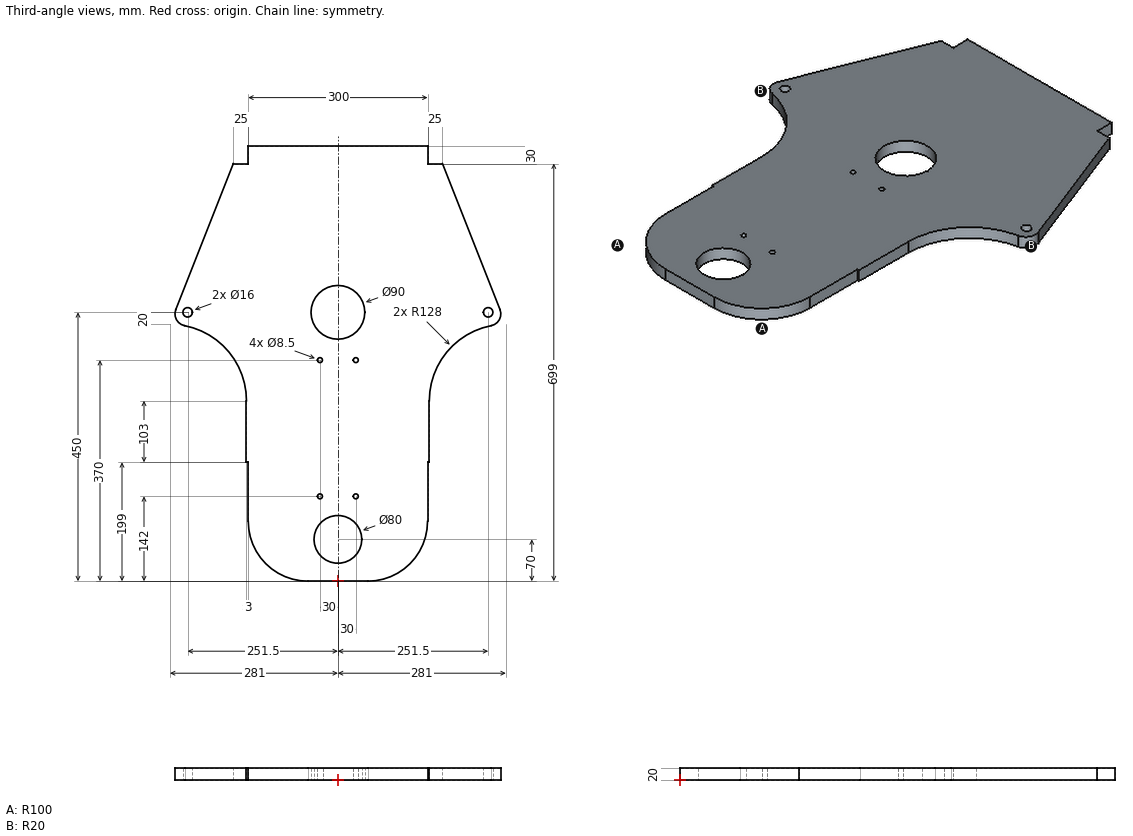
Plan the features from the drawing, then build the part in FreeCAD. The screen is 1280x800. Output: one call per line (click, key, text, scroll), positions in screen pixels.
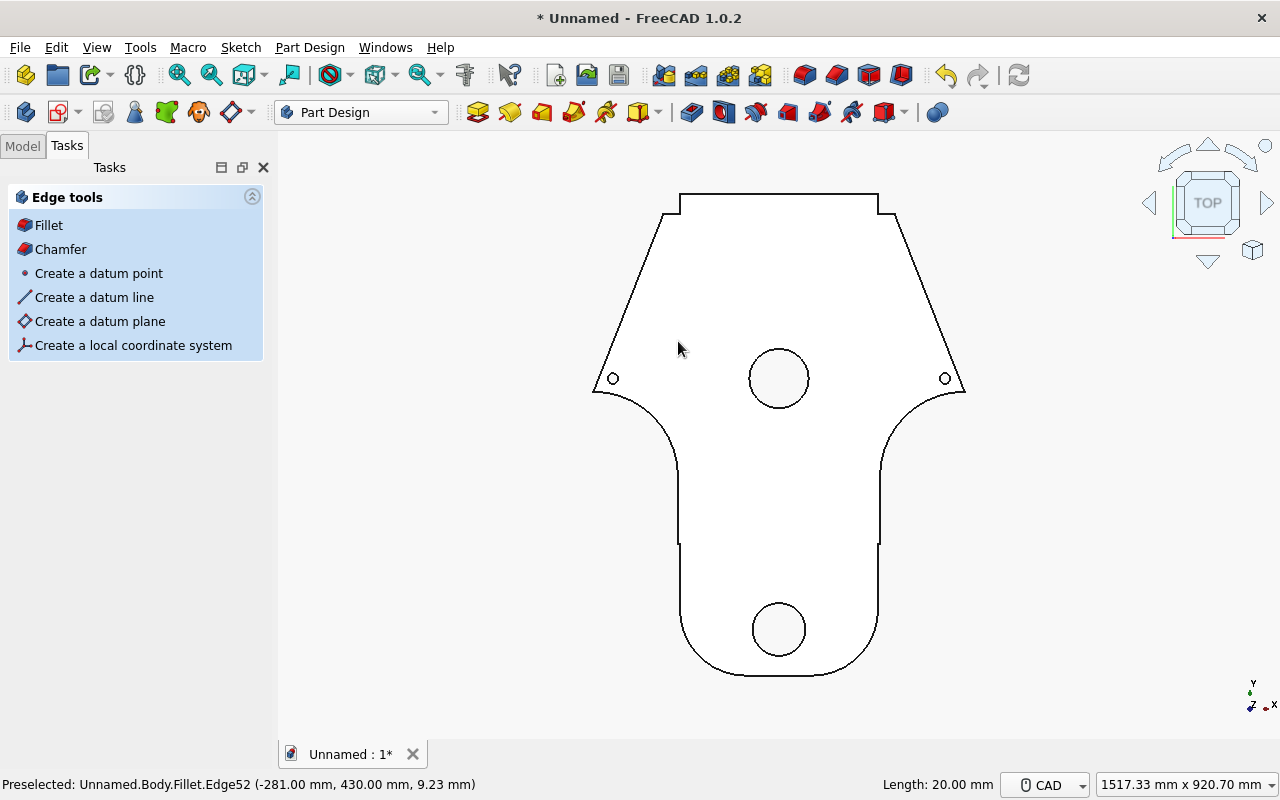
scroll(593, 391, up, 6)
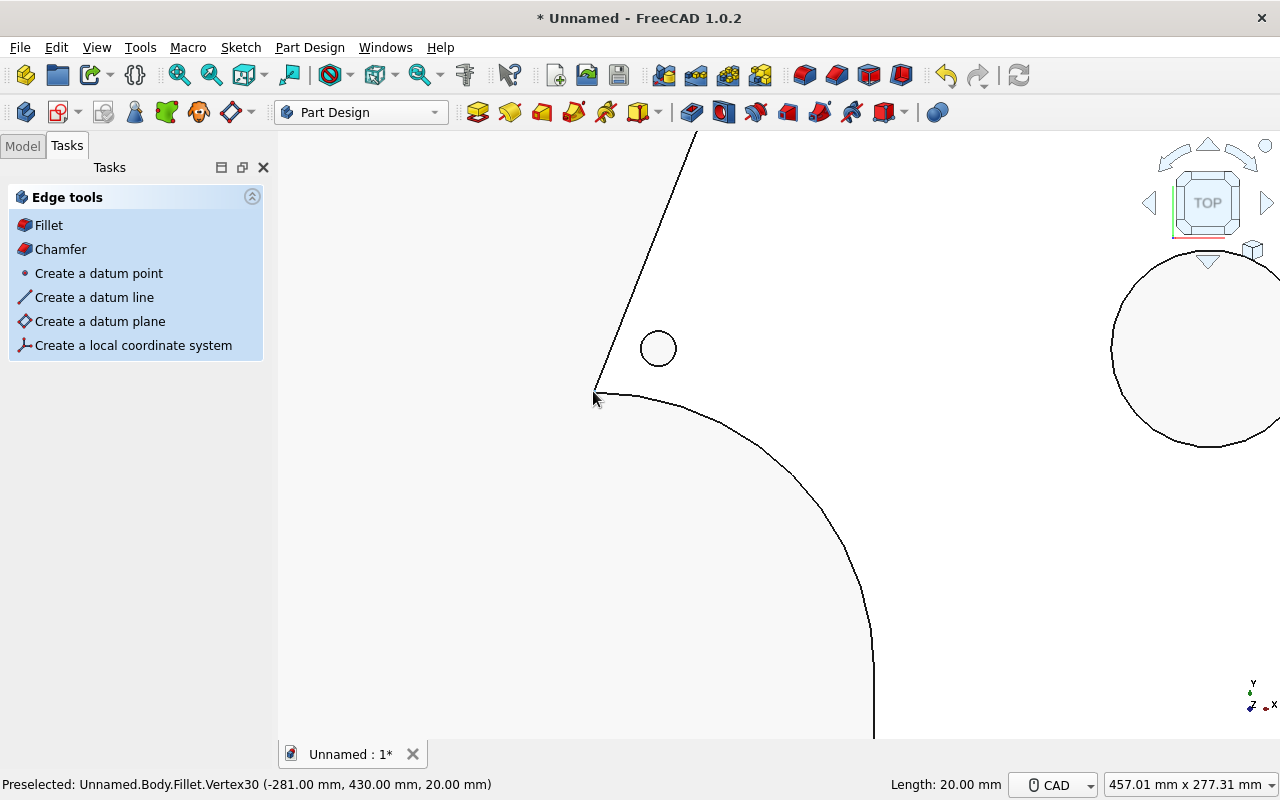
click(180, 76)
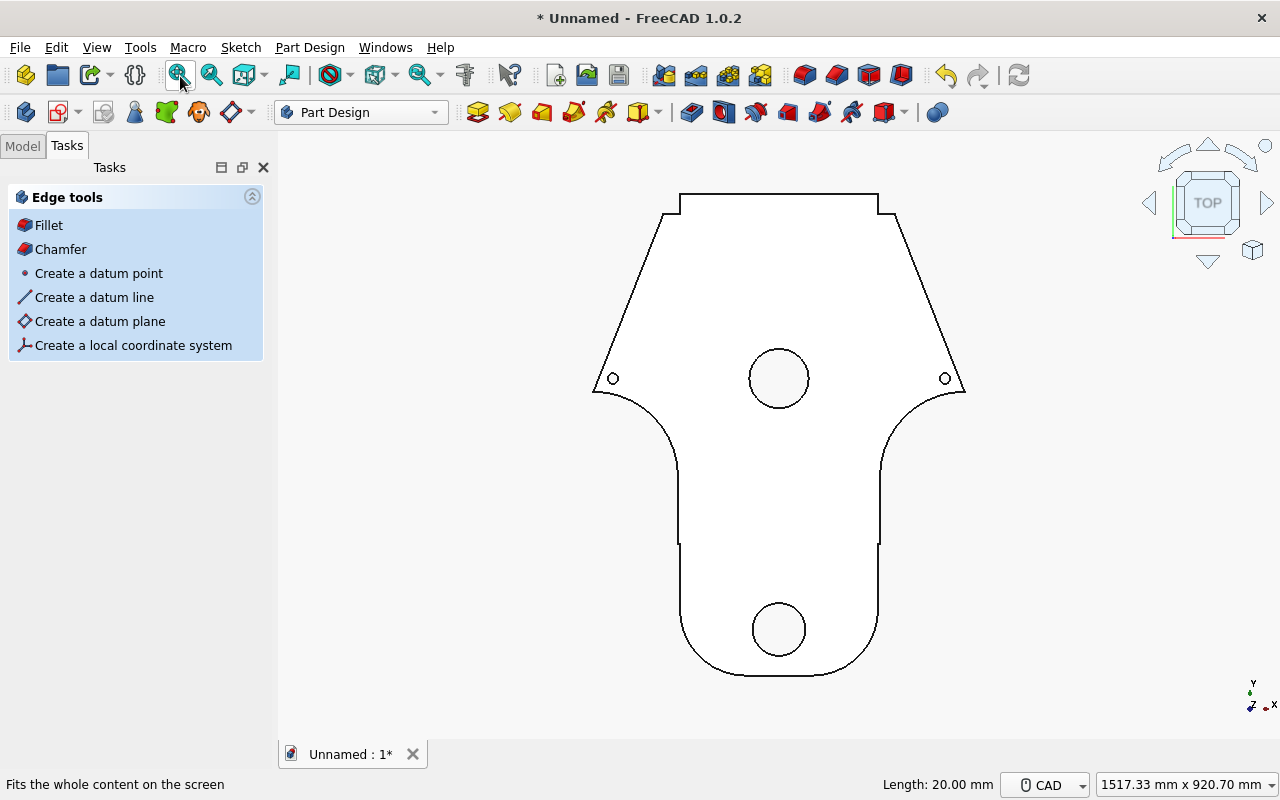
key(1)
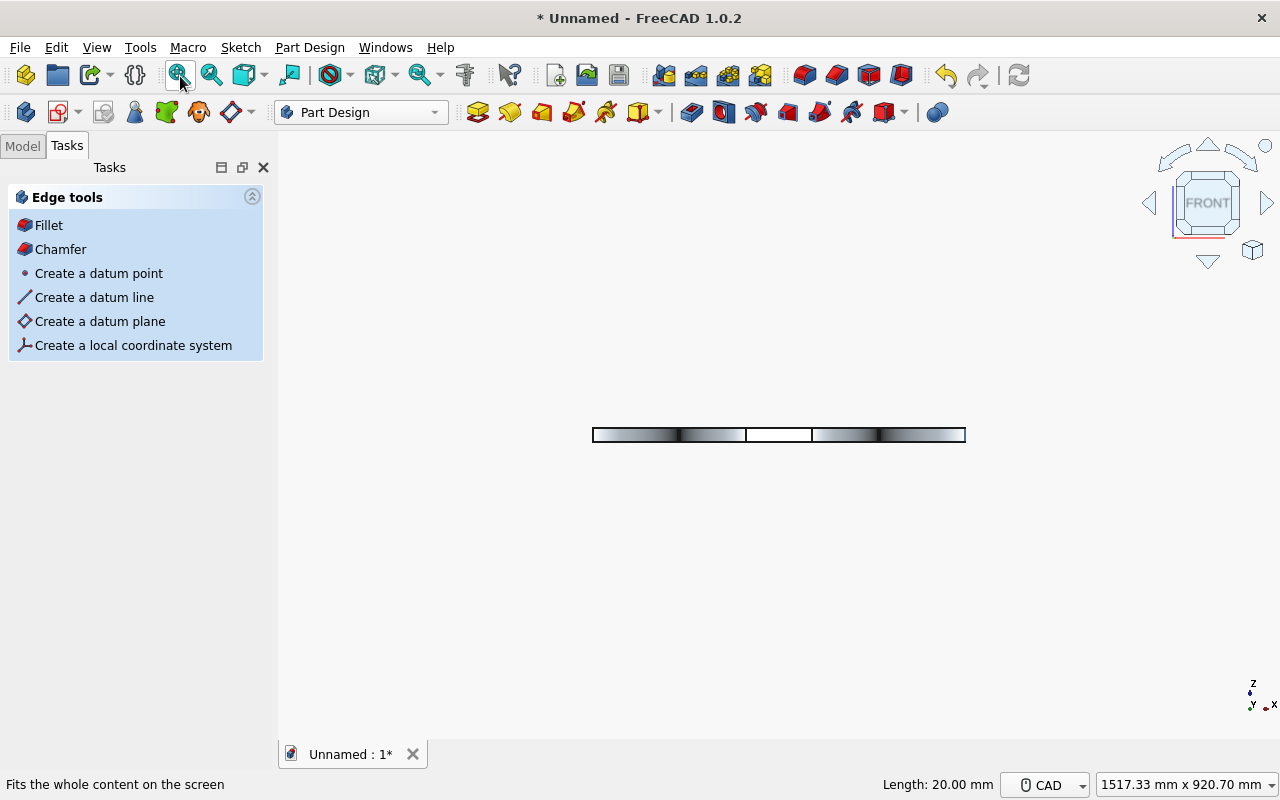
click(180, 76)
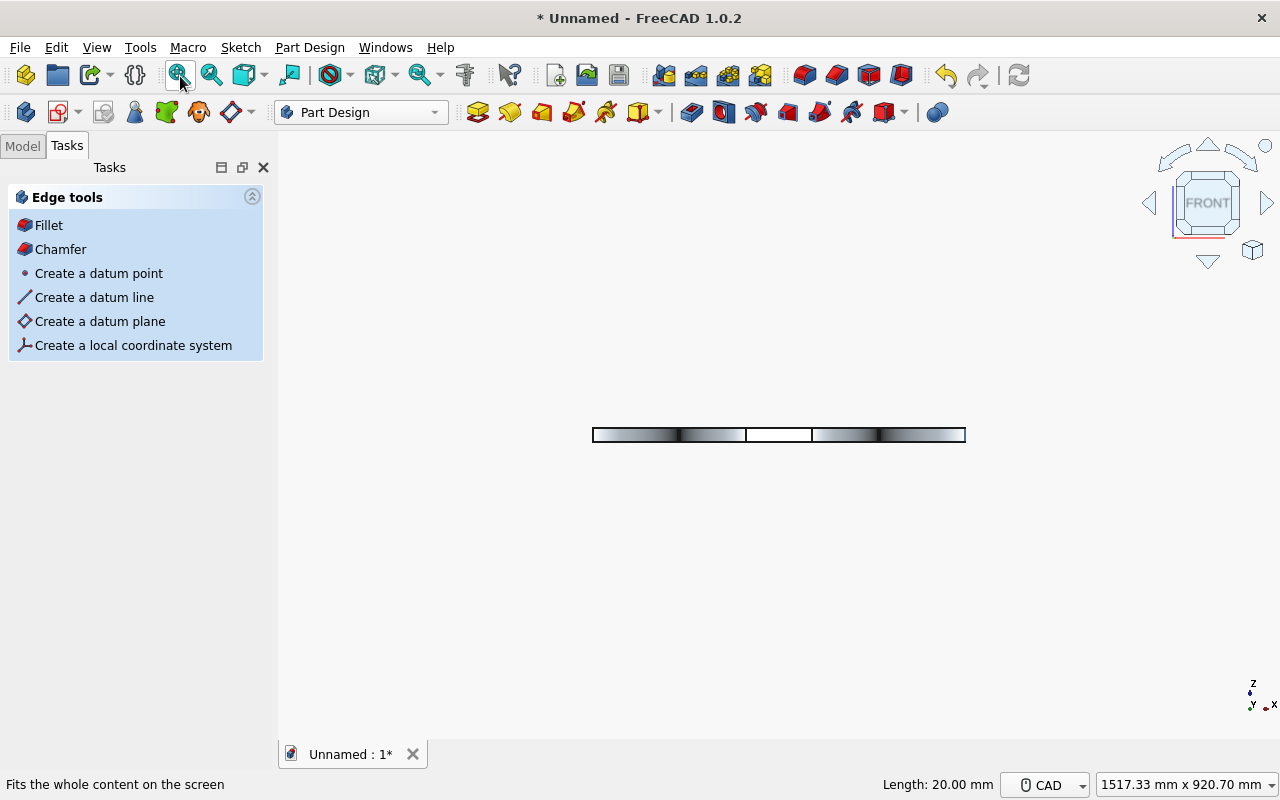
scroll(593, 434, up, 6)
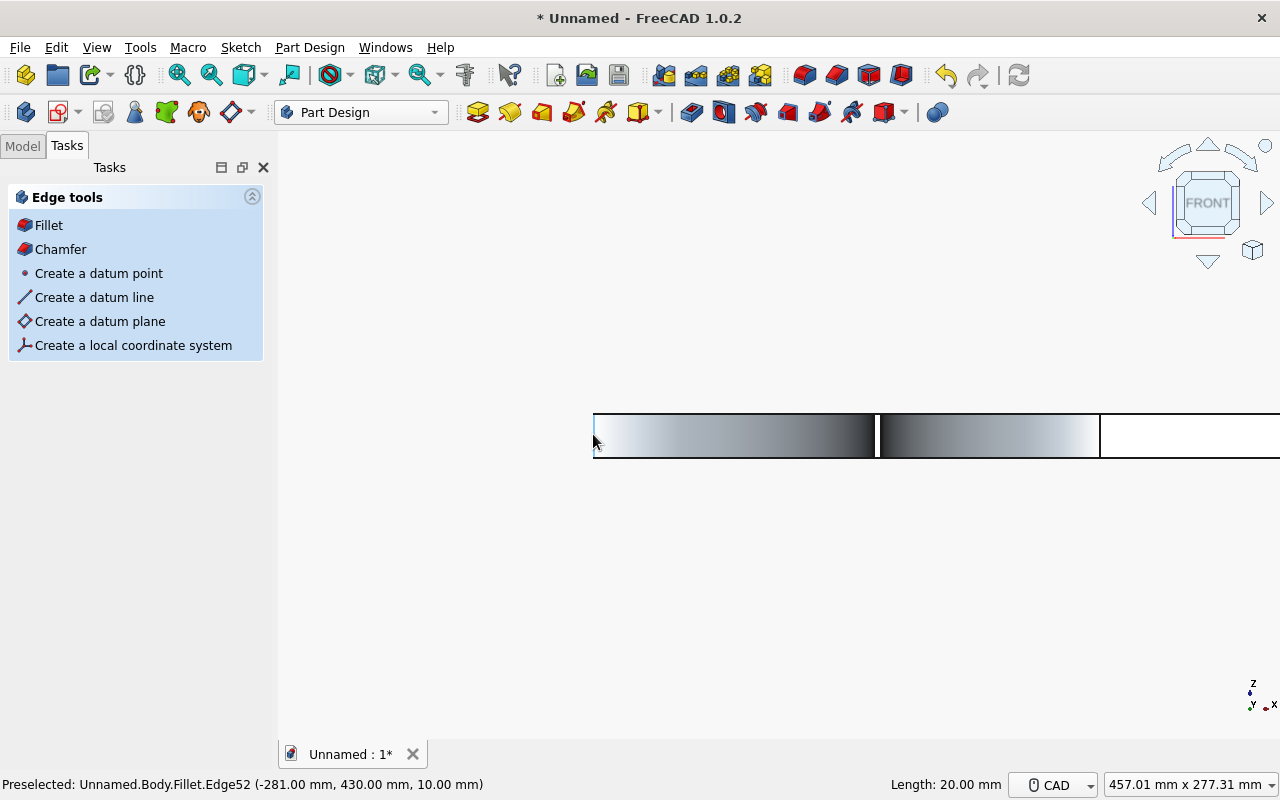
click(180, 76)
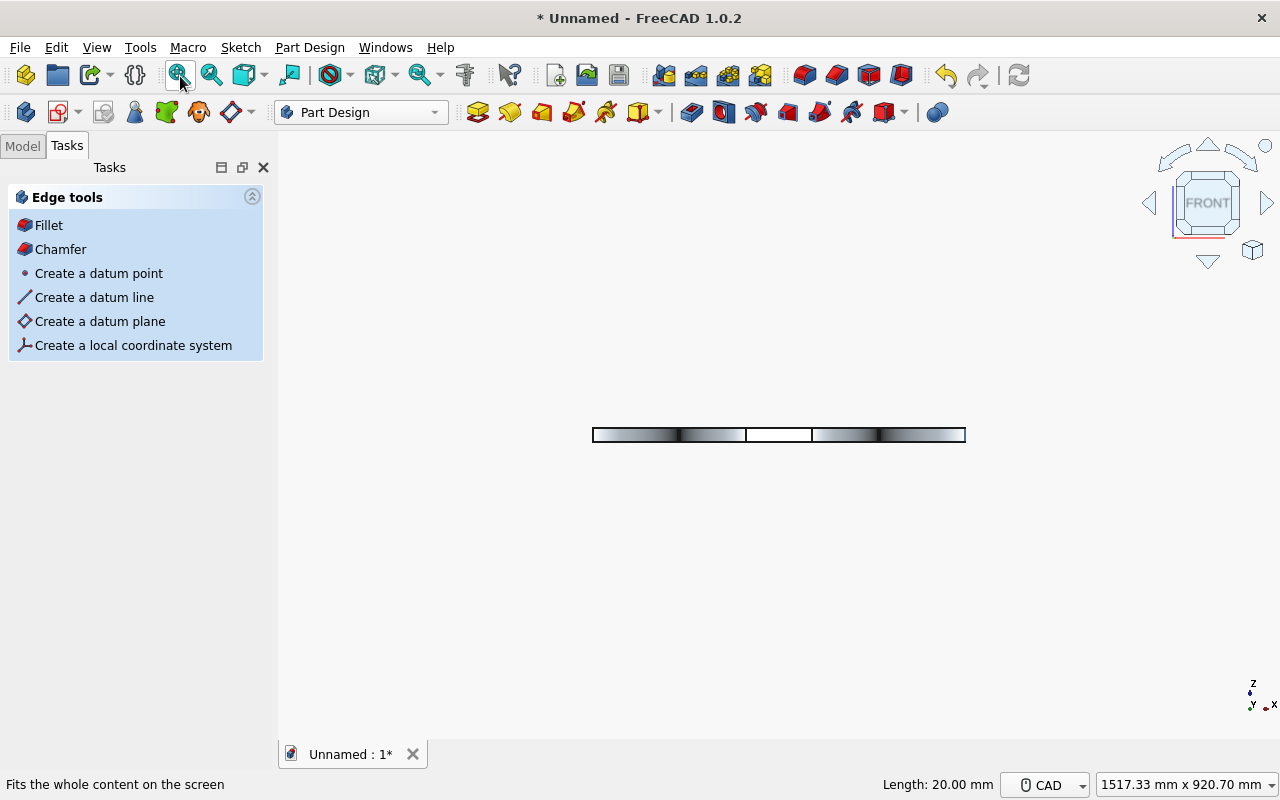
key(3)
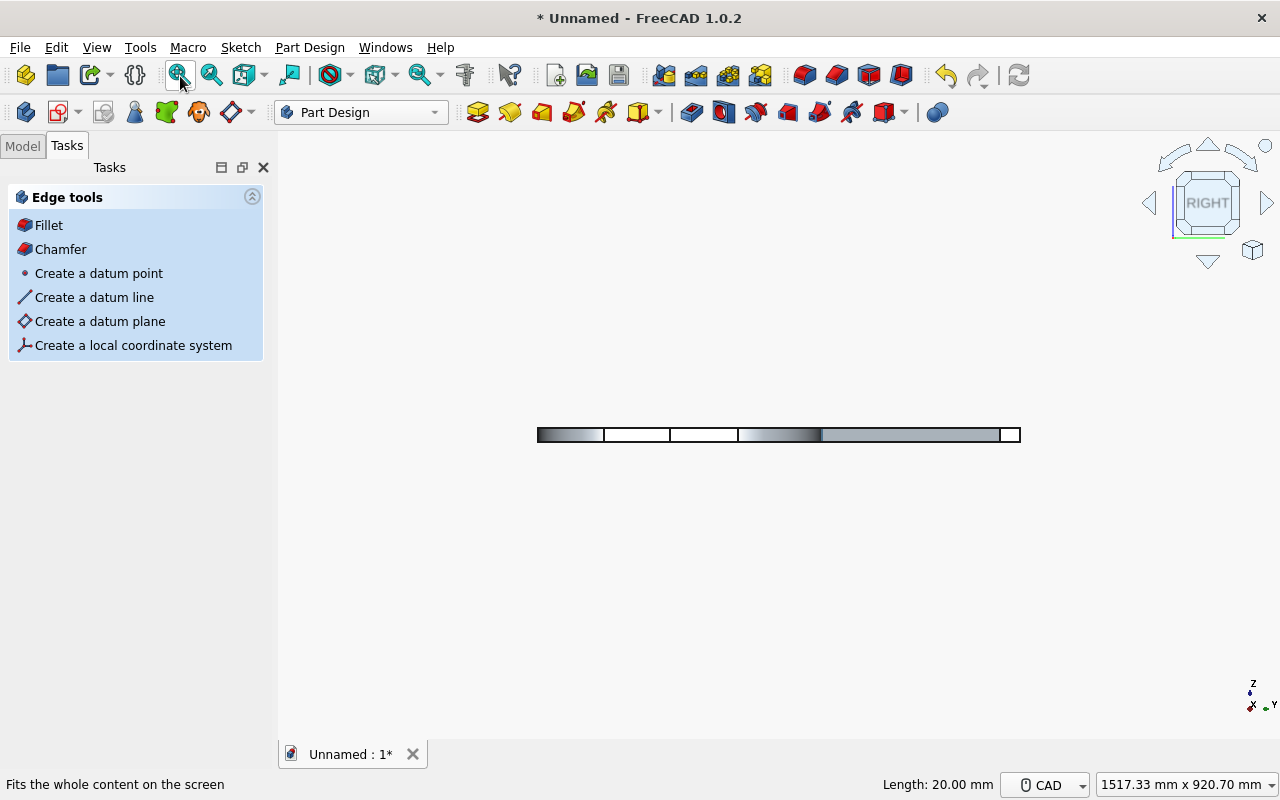
scroll(822, 434, up, 6)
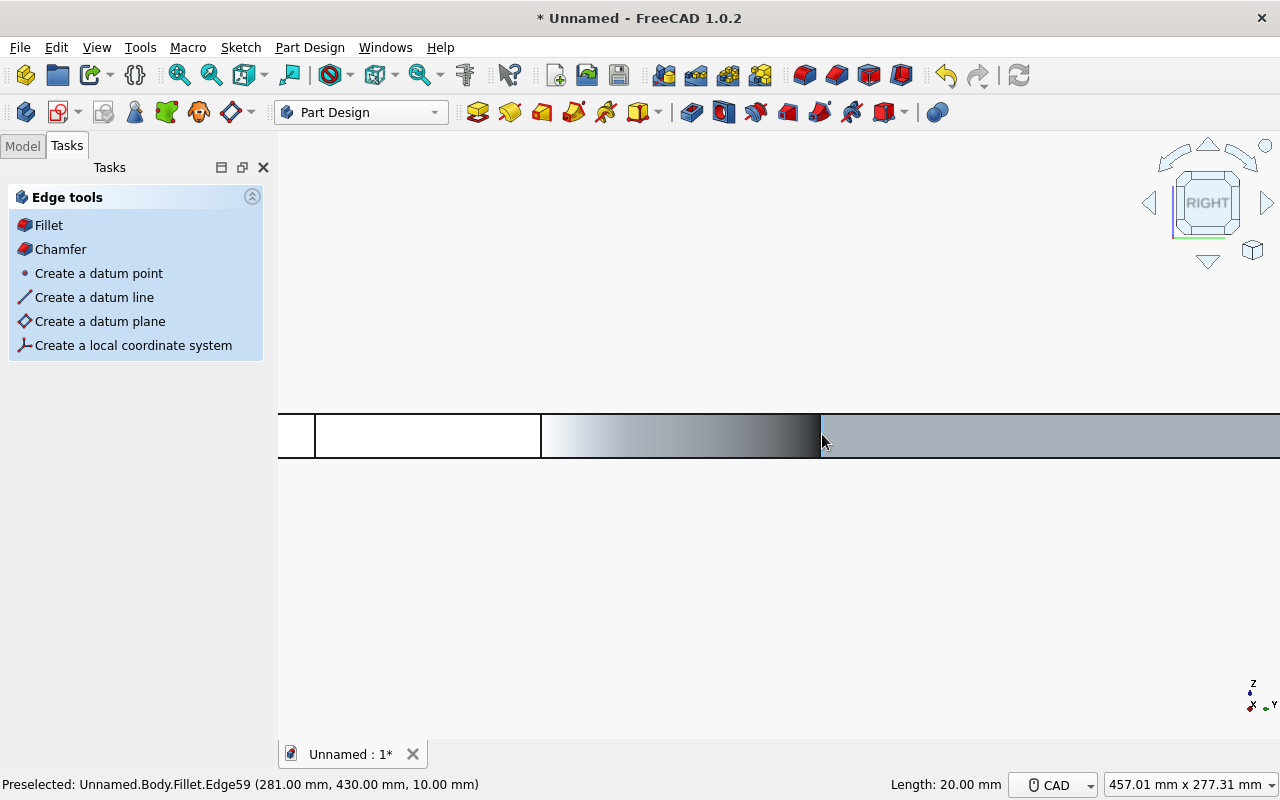
click(180, 76)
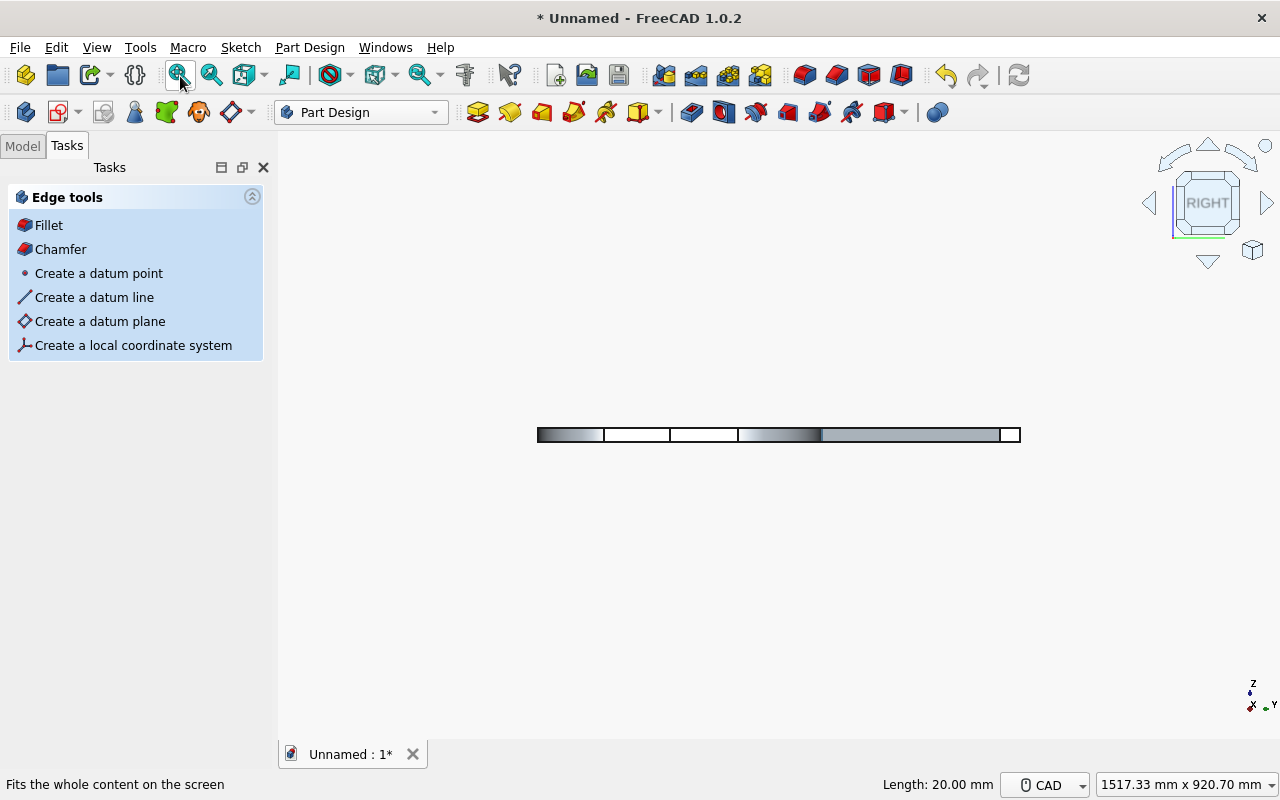
key(5)